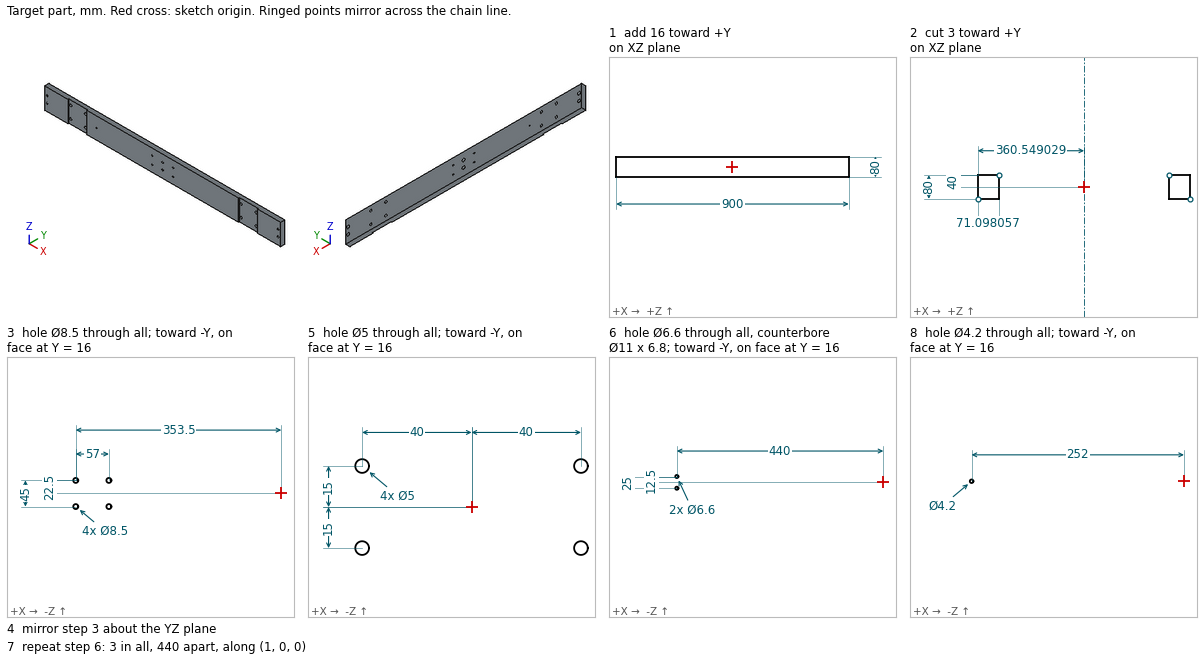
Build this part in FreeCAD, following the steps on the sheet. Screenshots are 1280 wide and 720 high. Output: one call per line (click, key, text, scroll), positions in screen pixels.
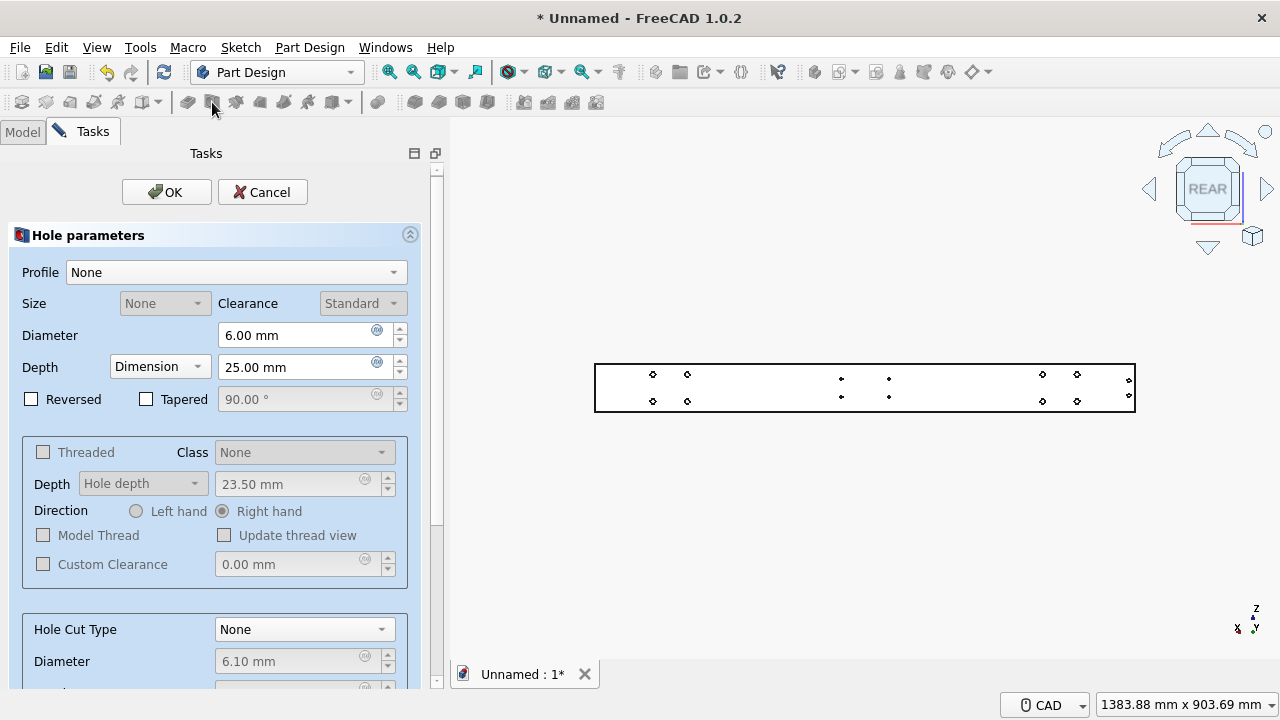
triple_click(305, 335)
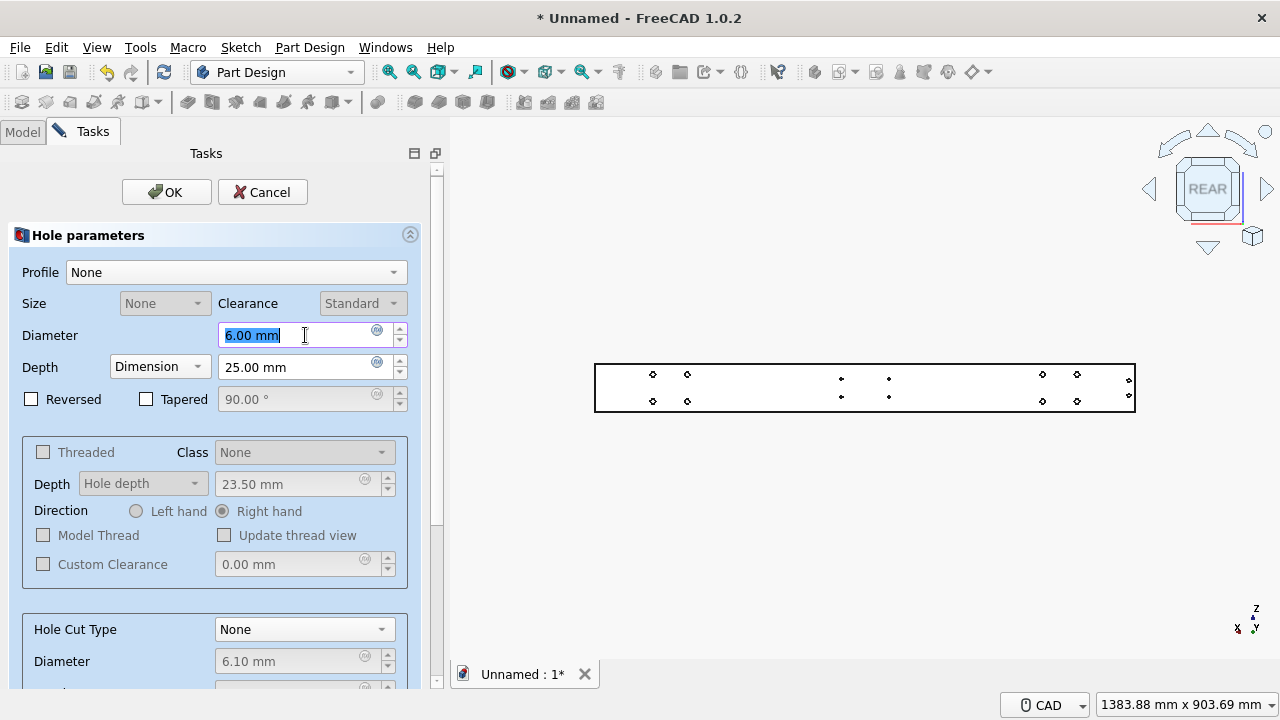
text(6.6)
key(Tab)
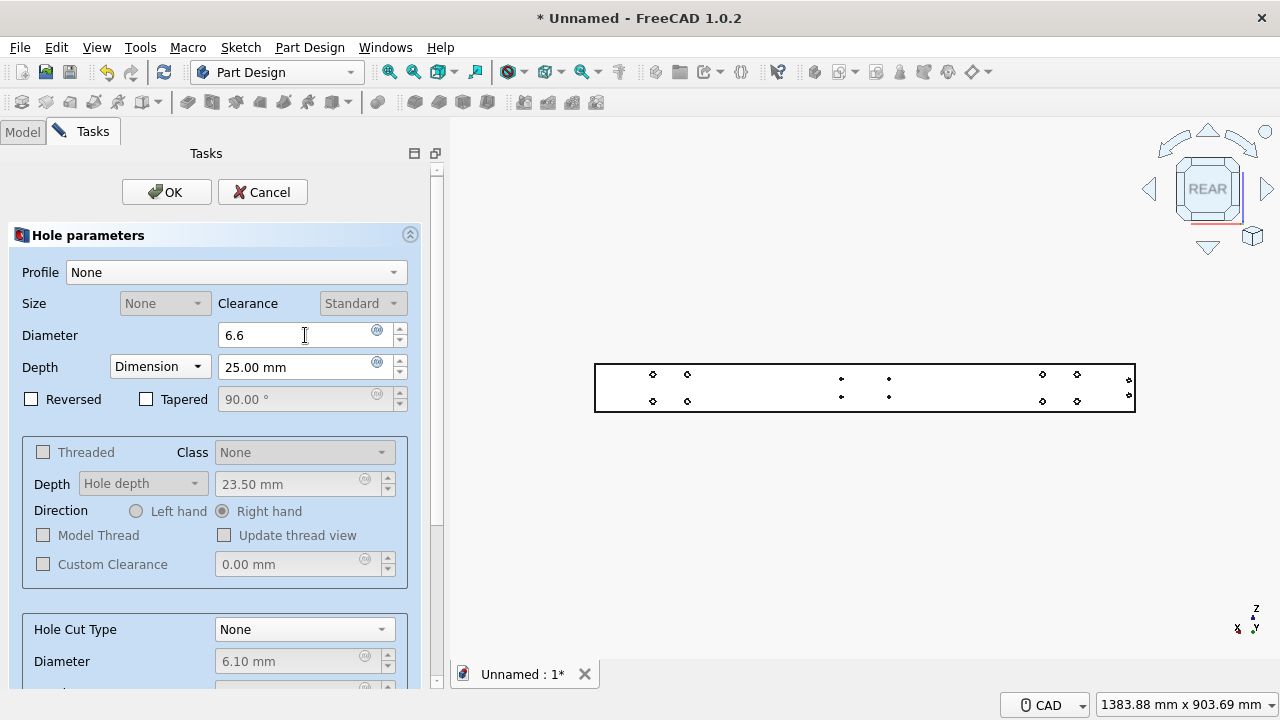
click(161, 366)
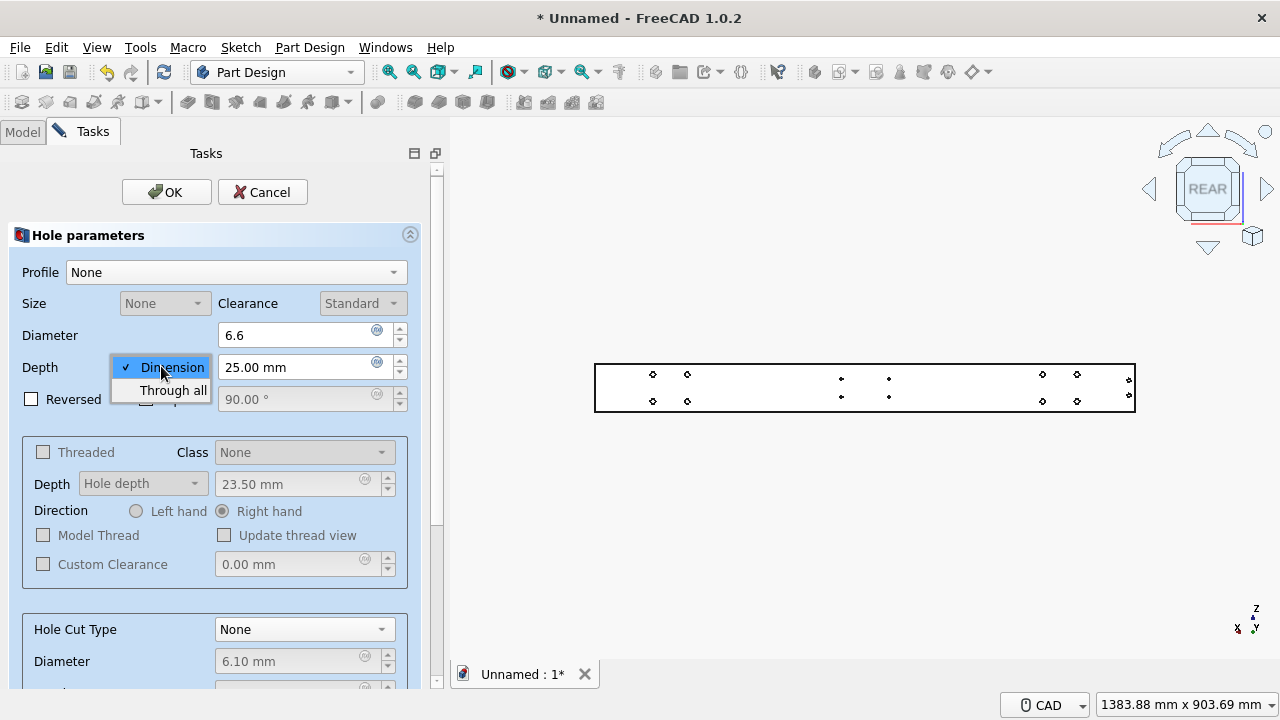
click(160, 390)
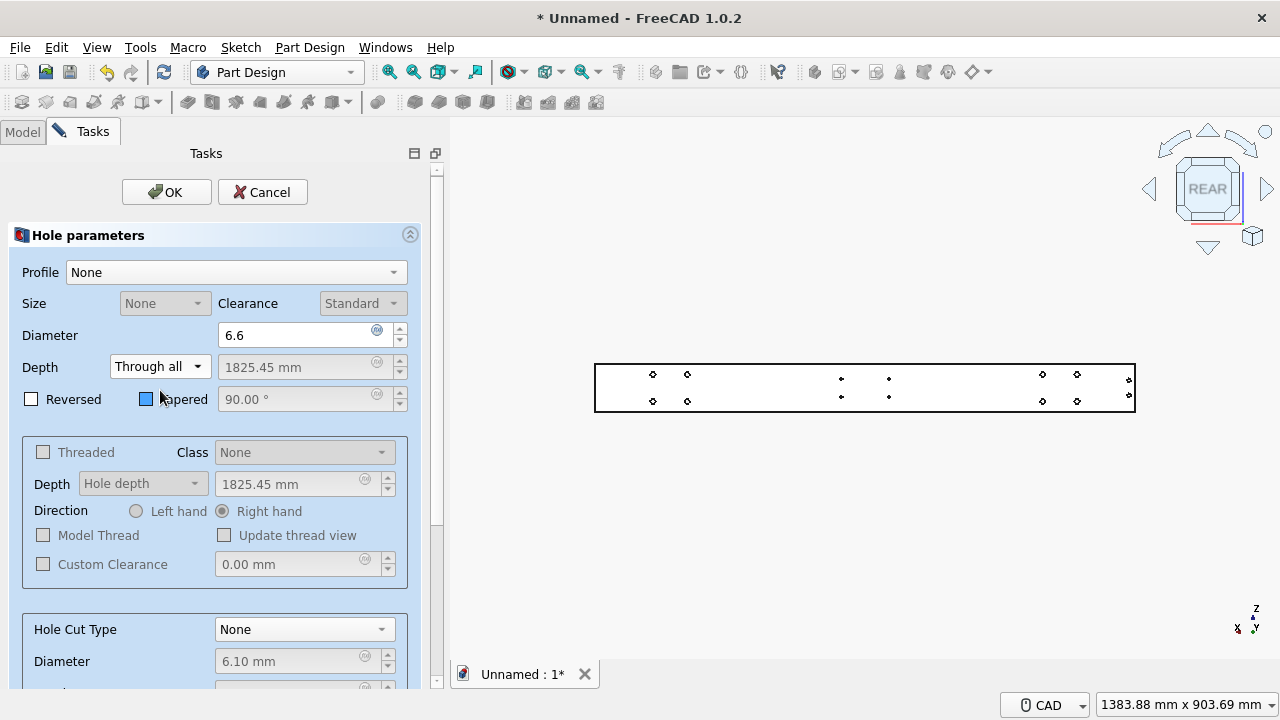
click(306, 630)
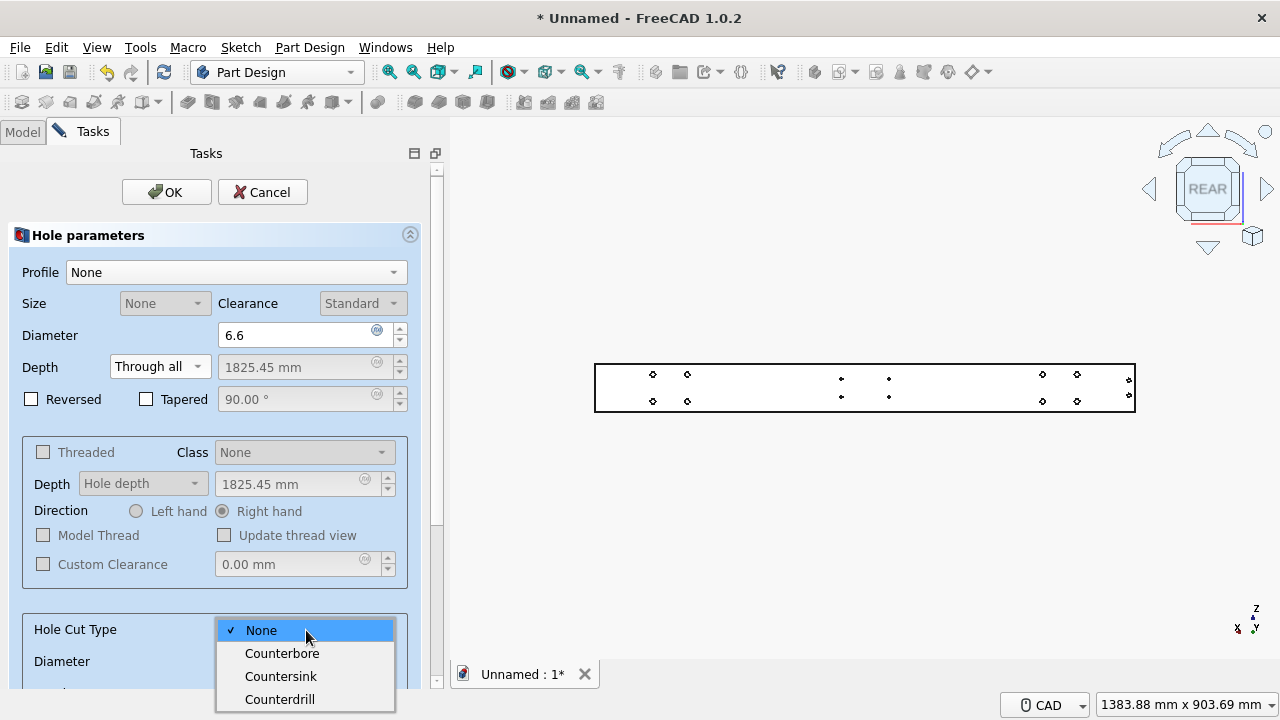
click(304, 654)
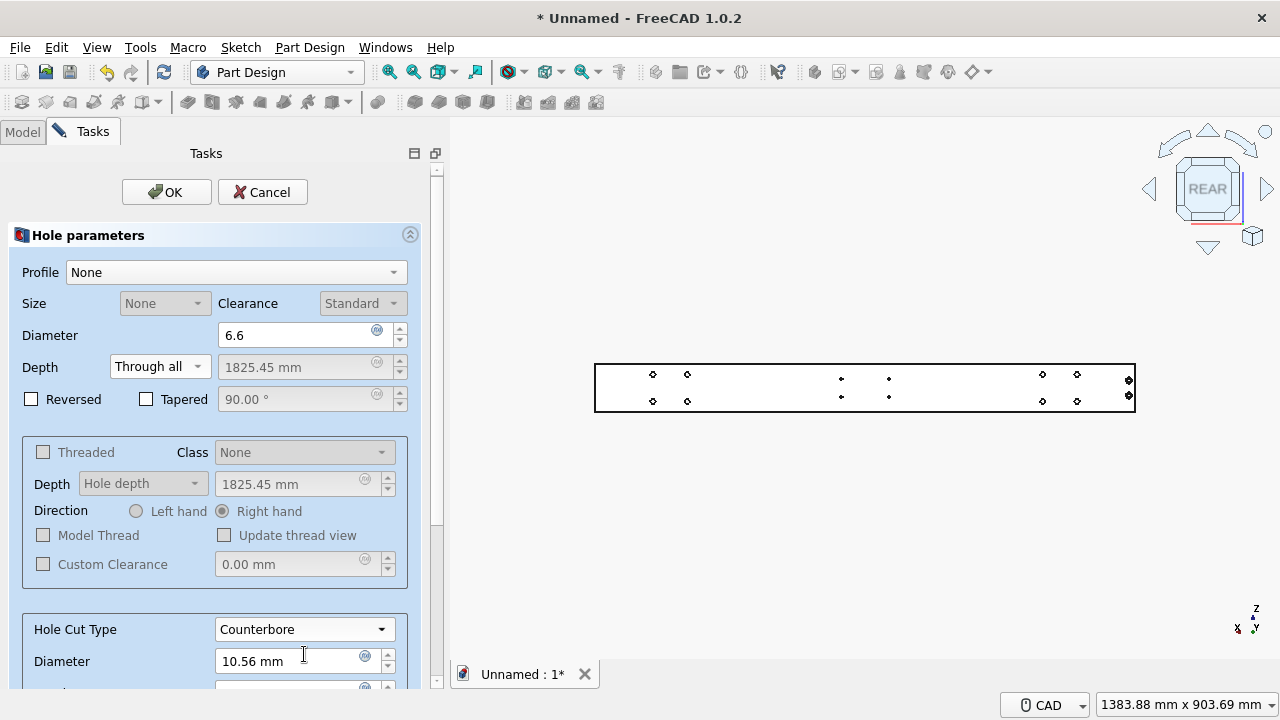
triple_click(298, 661)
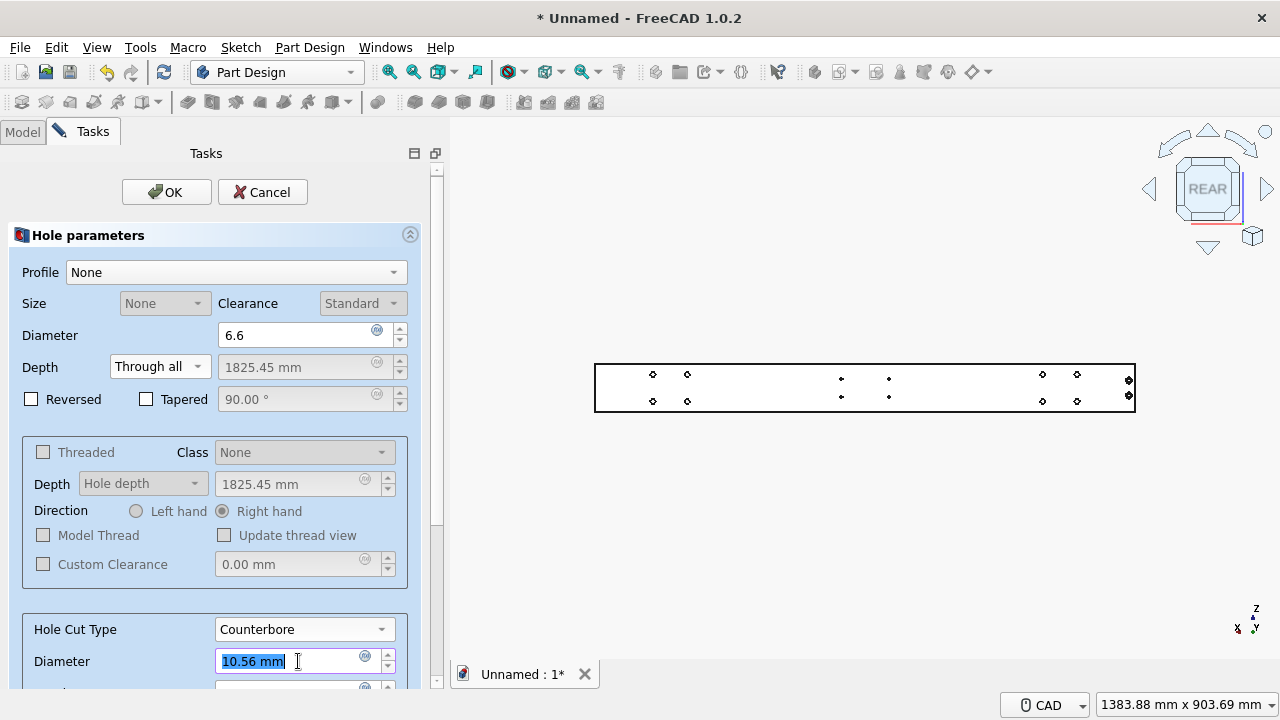
text(11)
key(Tab)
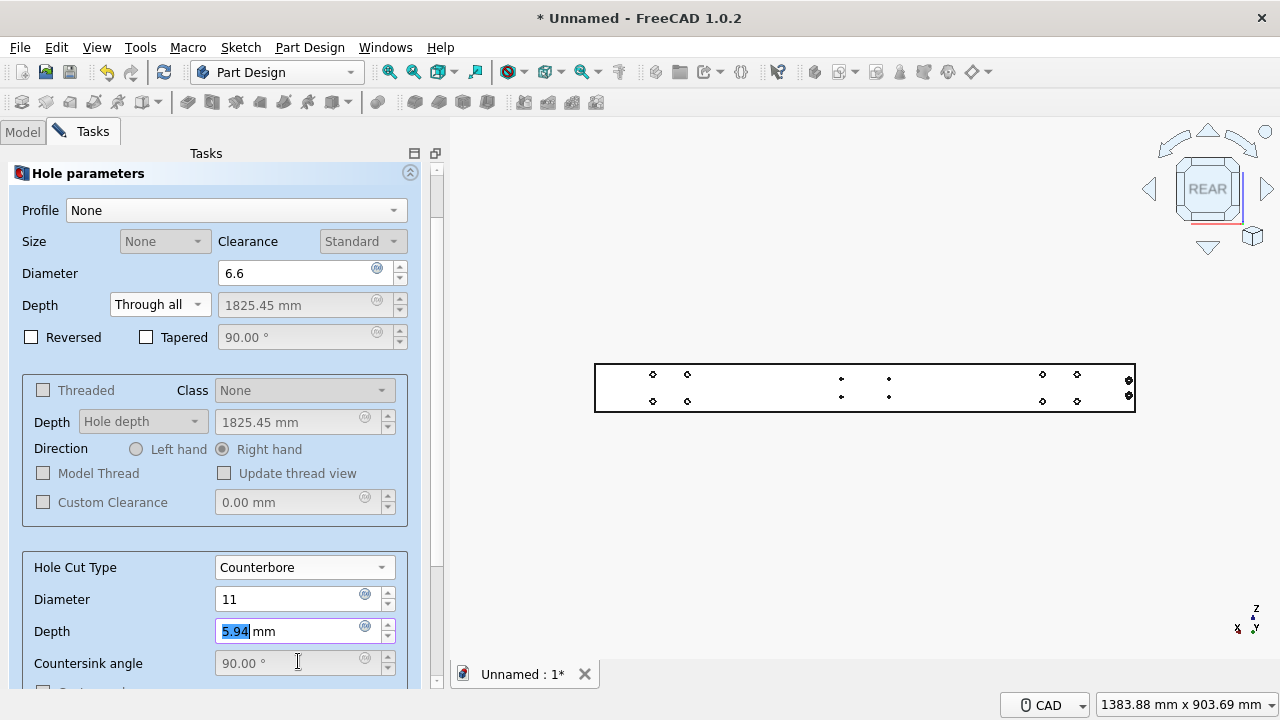
text(6.8)
key(Tab)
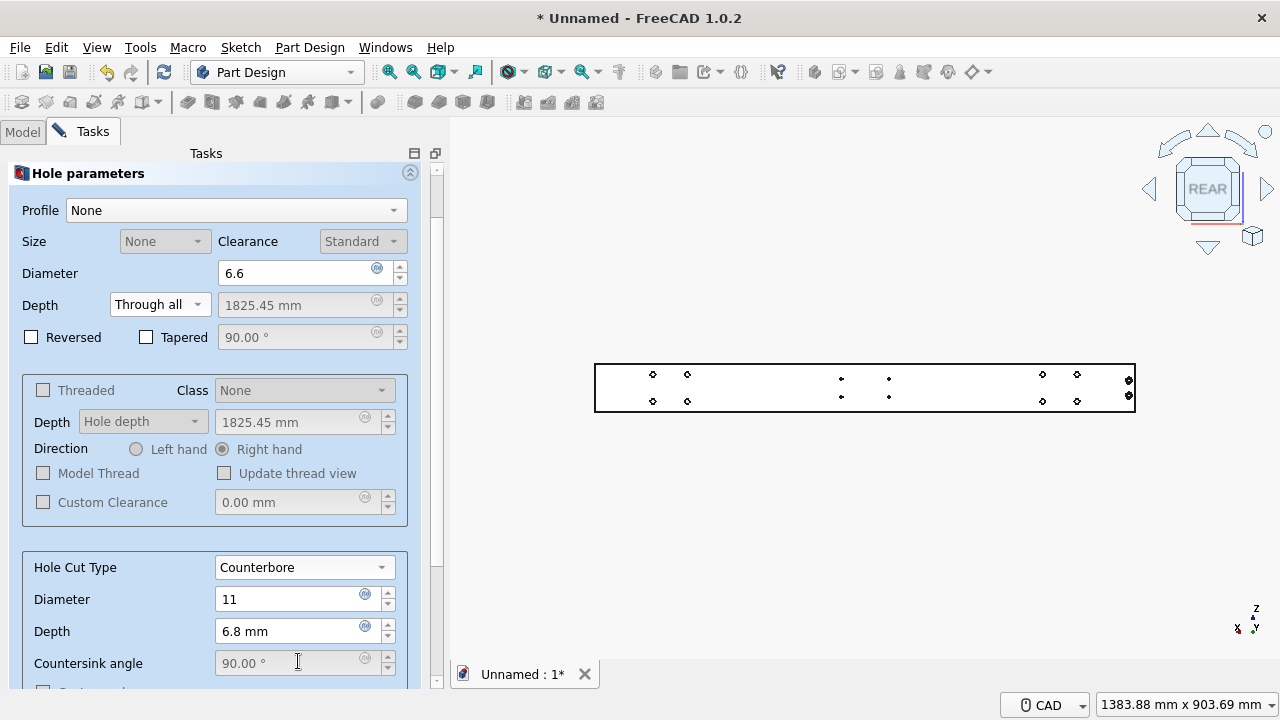
scroll(437, 426, up, 2)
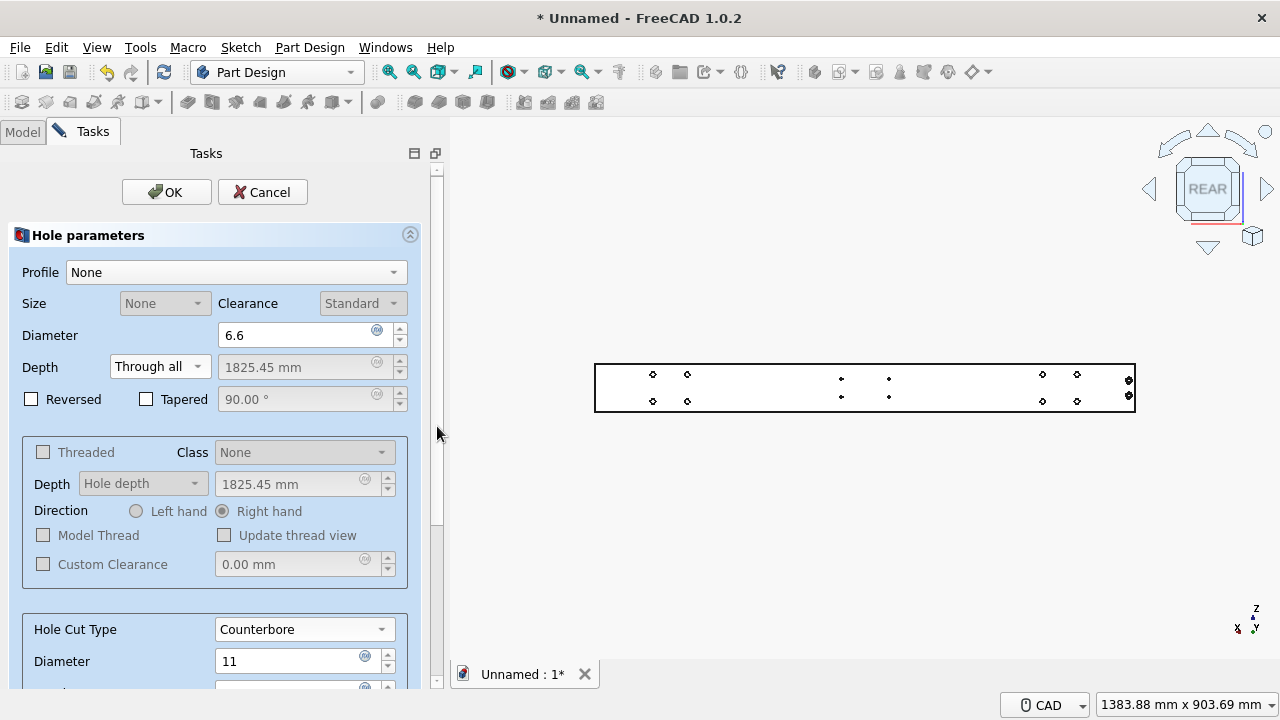
click(167, 192)